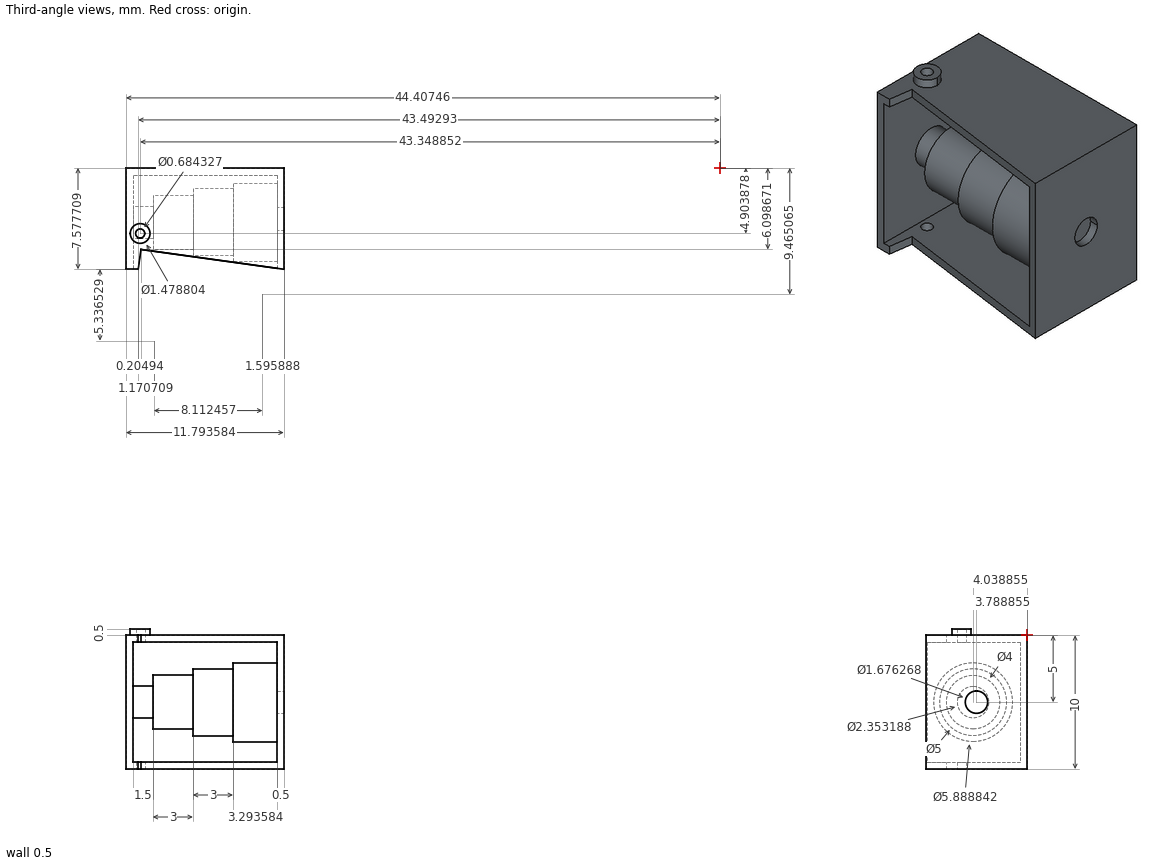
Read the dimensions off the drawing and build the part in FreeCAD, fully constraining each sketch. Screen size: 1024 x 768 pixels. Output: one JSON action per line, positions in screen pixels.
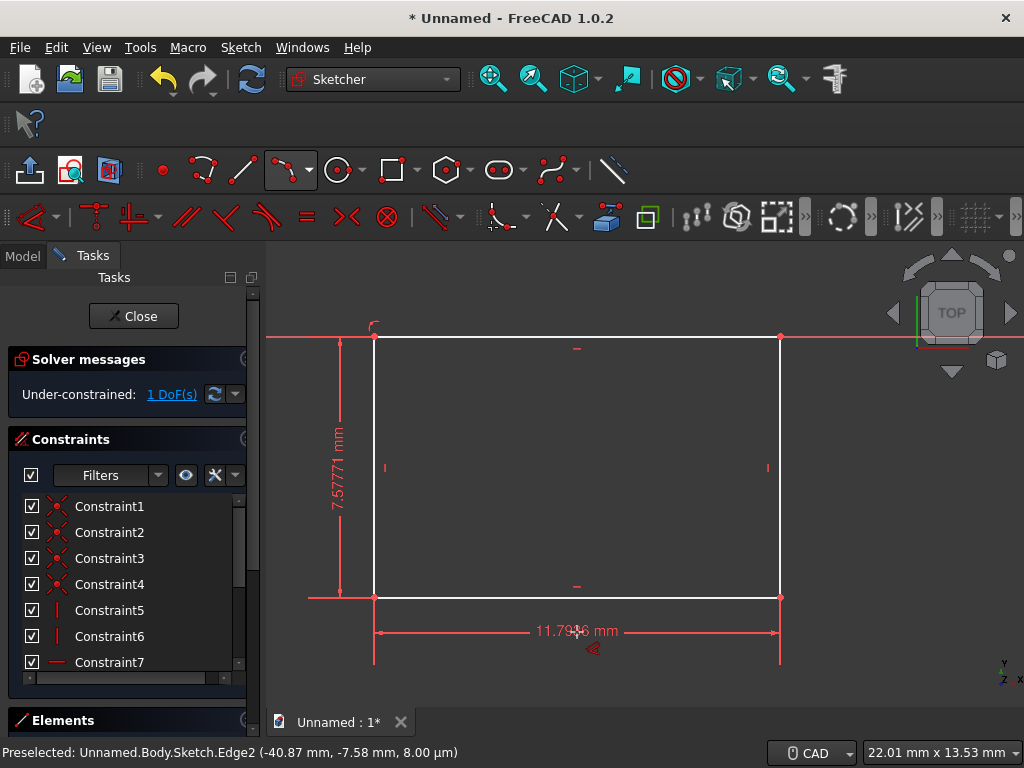
{"action": "left_click", "coordinate": [374, 337]}
{"action": "left_click", "coordinate": [617, 303]}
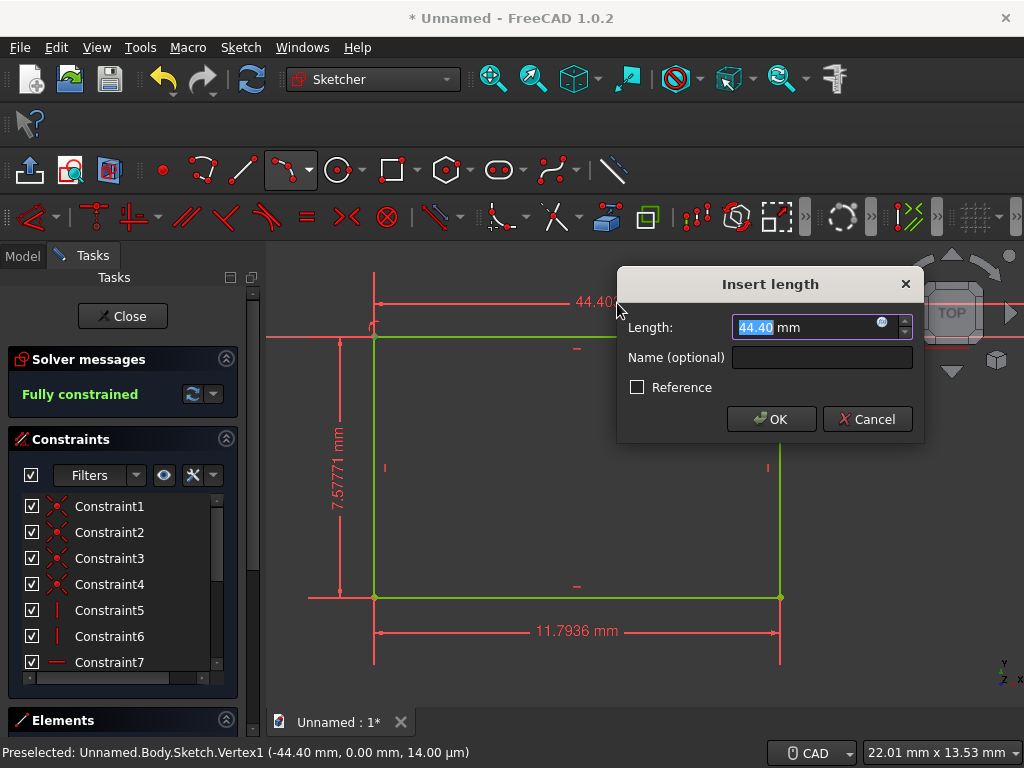
{"action": "type", "text": "44.40746"}
{"action": "key", "text": "Return"}
{"action": "key", "text": "Escape"}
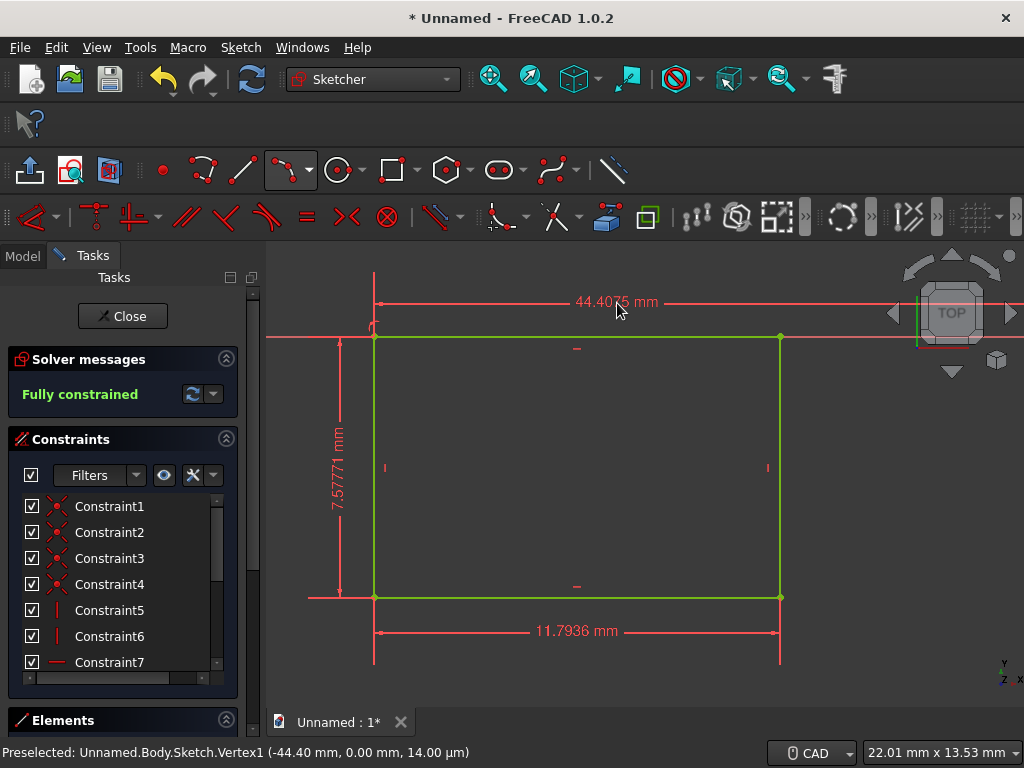
{"action": "left_click", "coordinate": [123, 316]}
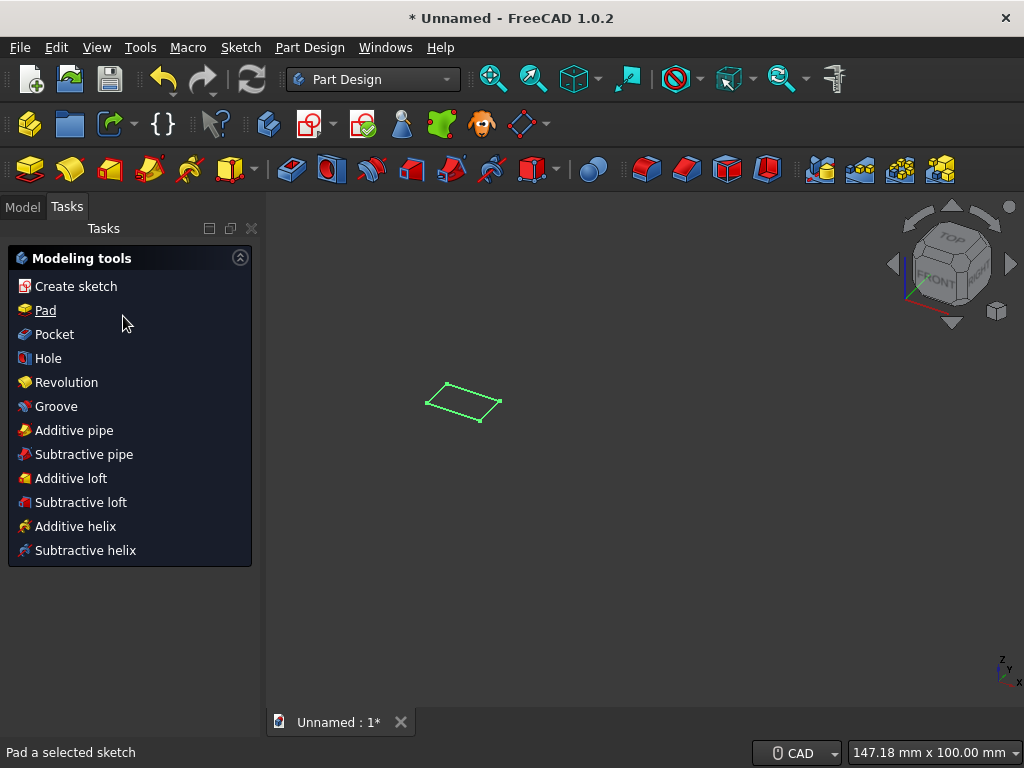
{"action": "left_click", "coordinate": [30, 170]}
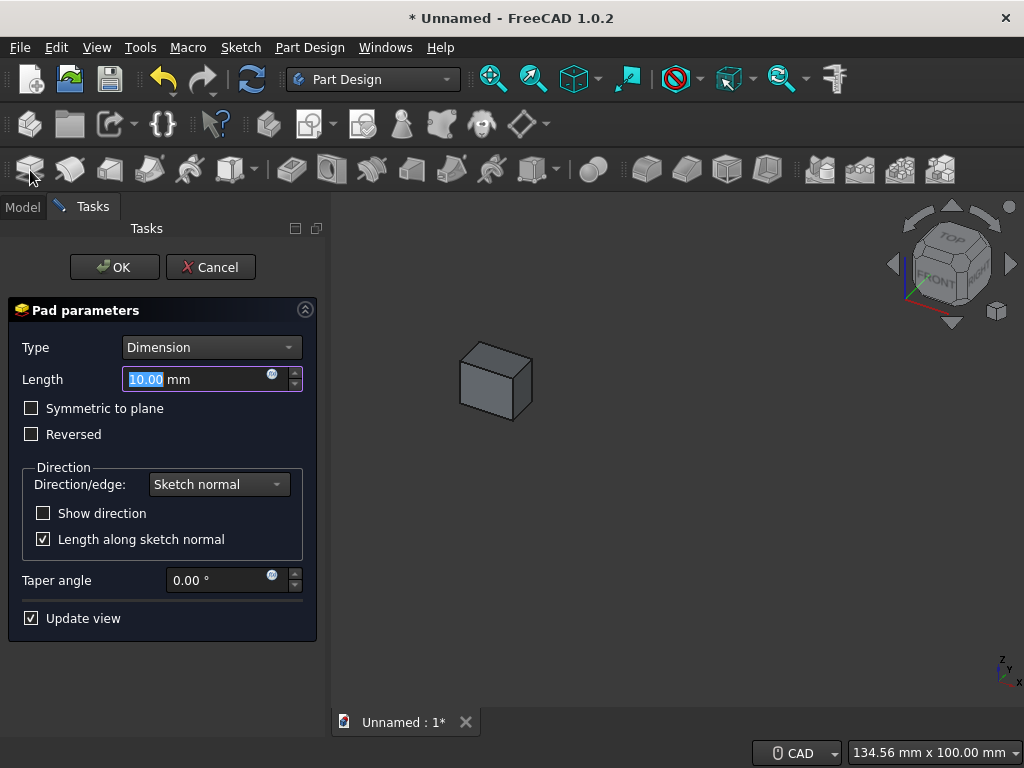
{"action": "type", "text": "10"}
{"action": "key", "text": "Tab"}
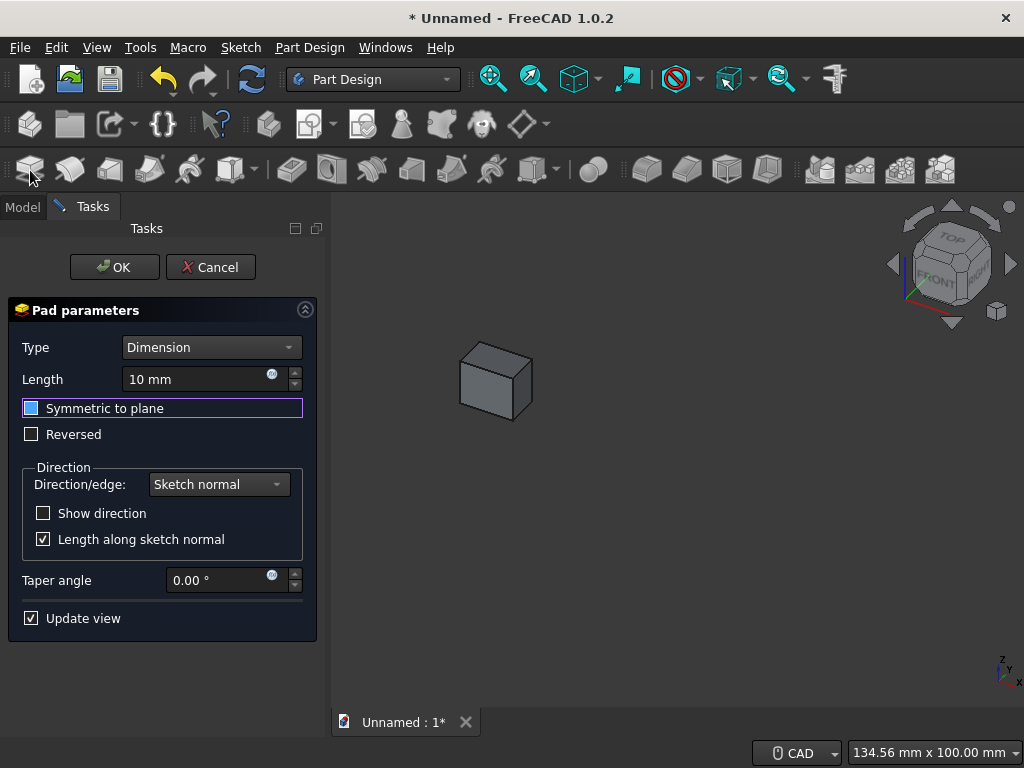
{"action": "left_click", "coordinate": [30, 434]}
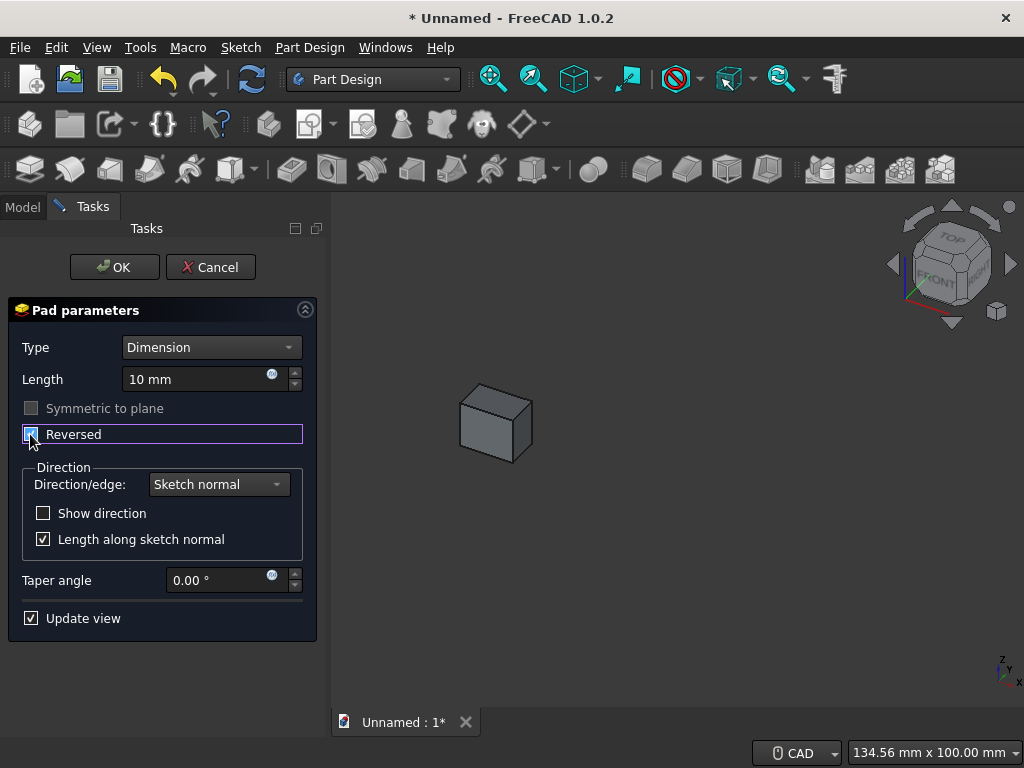
{"action": "left_click", "coordinate": [115, 267]}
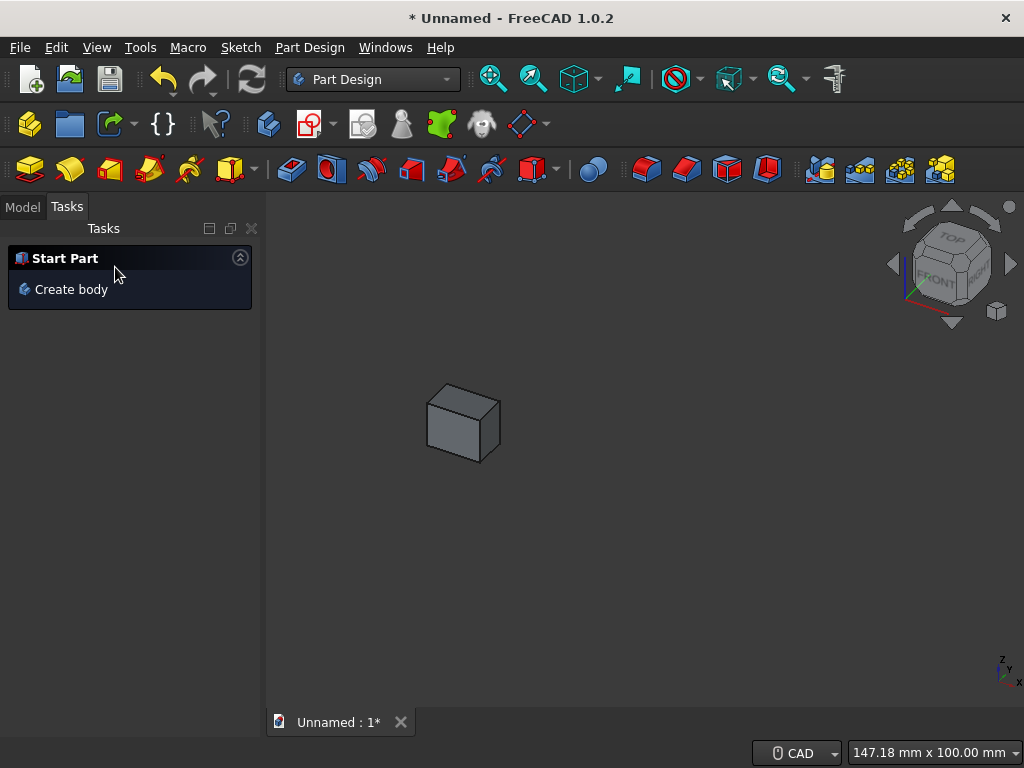
{"action": "left_click", "coordinate": [494, 80]}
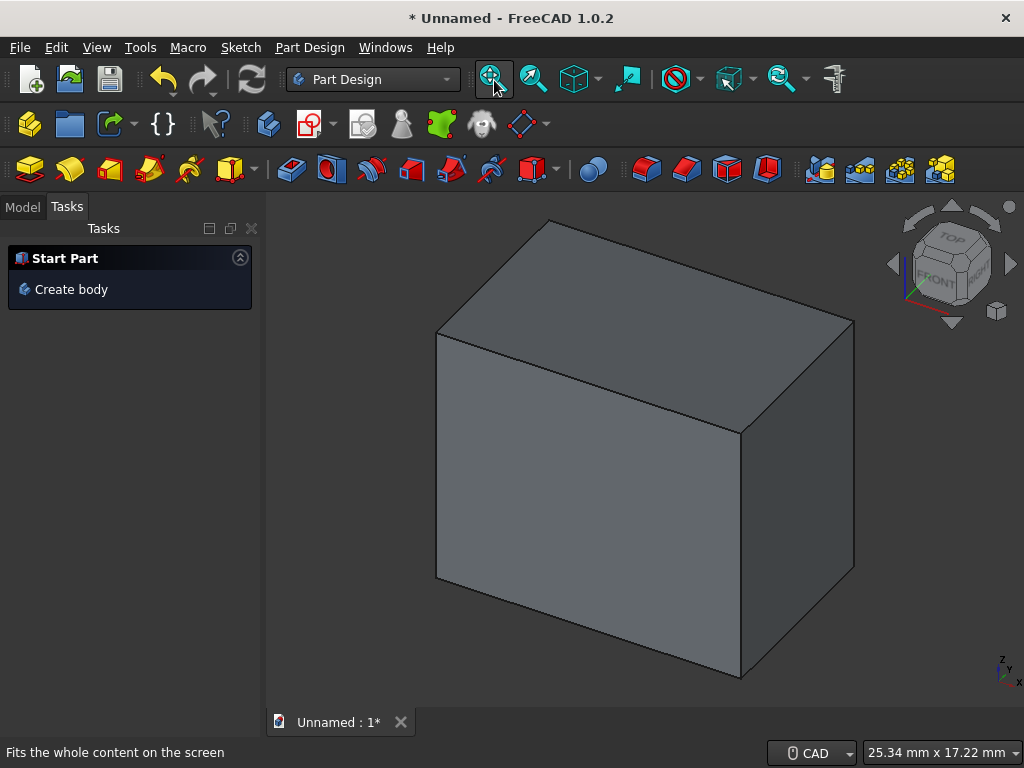
{"action": "left_click", "coordinate": [588, 505]}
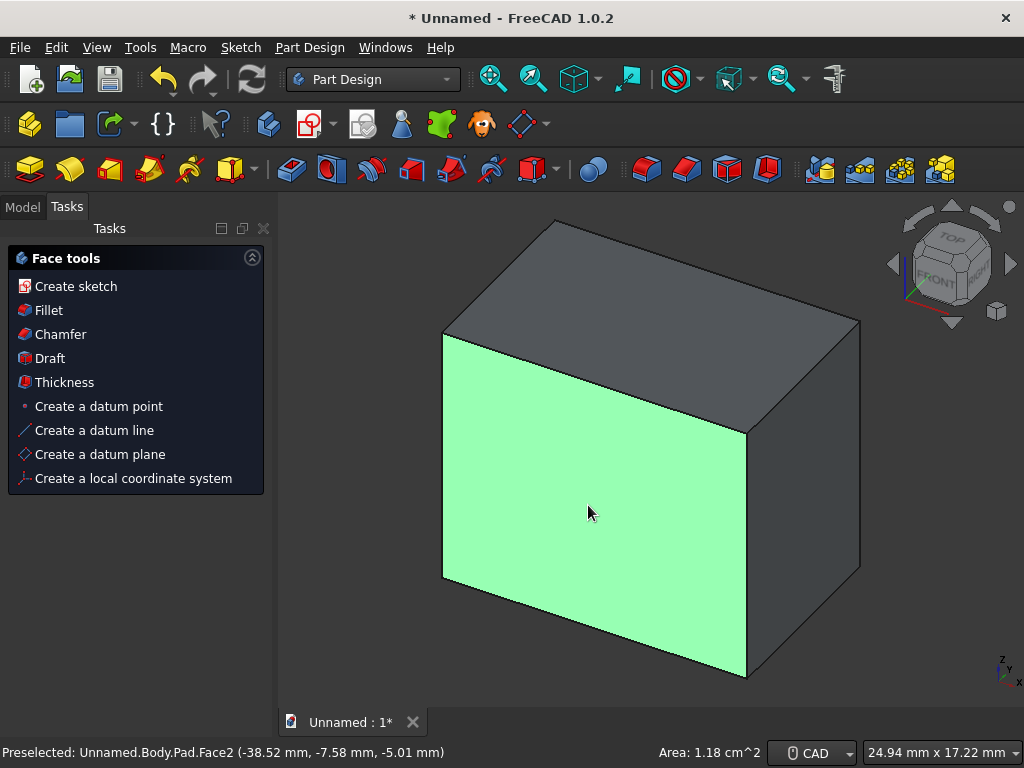
{"action": "left_click", "coordinate": [768, 170]}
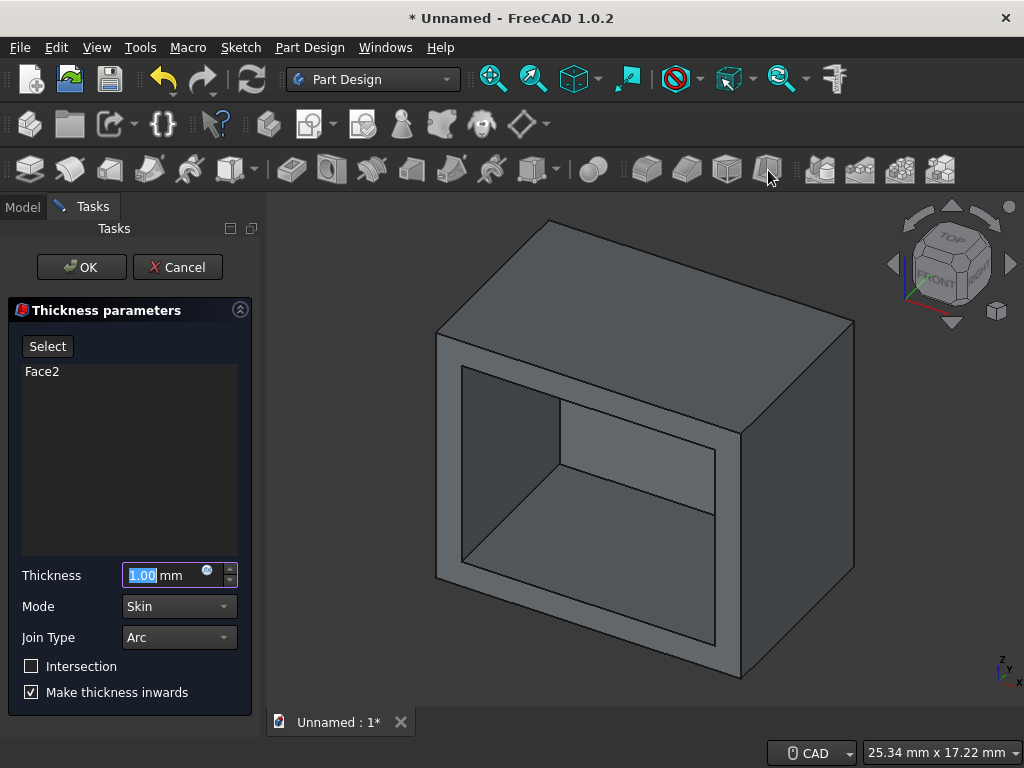
{"action": "type", "text": "0.5"}
{"action": "key", "text": "Tab"}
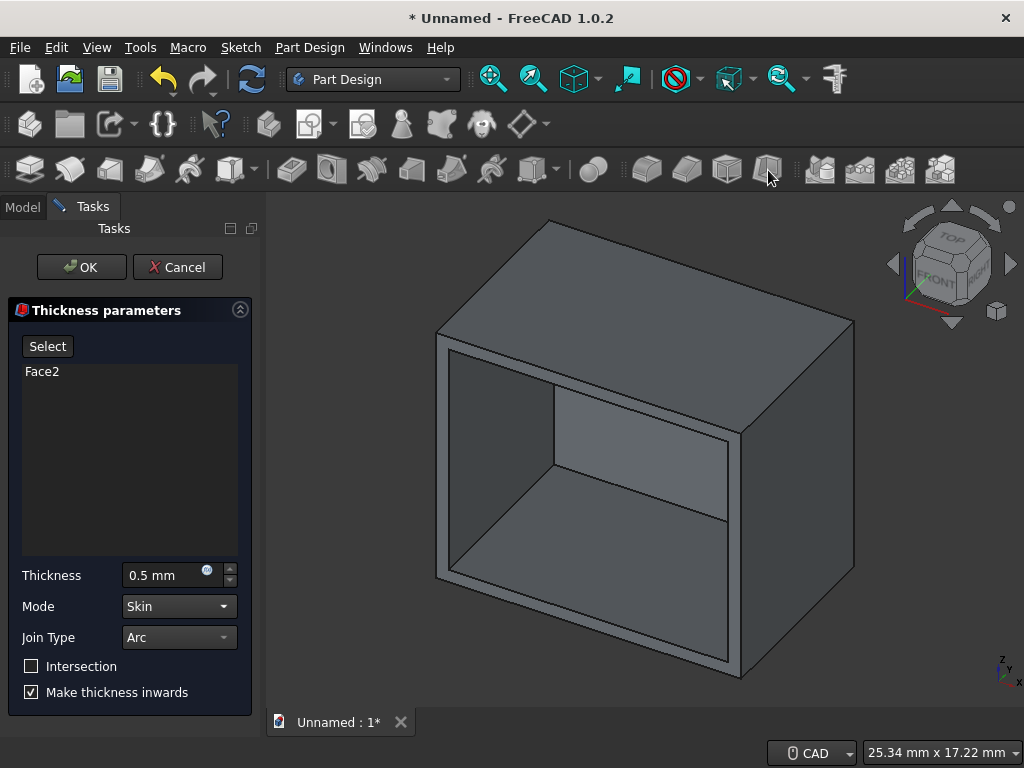
{"action": "left_click", "coordinate": [180, 638]}